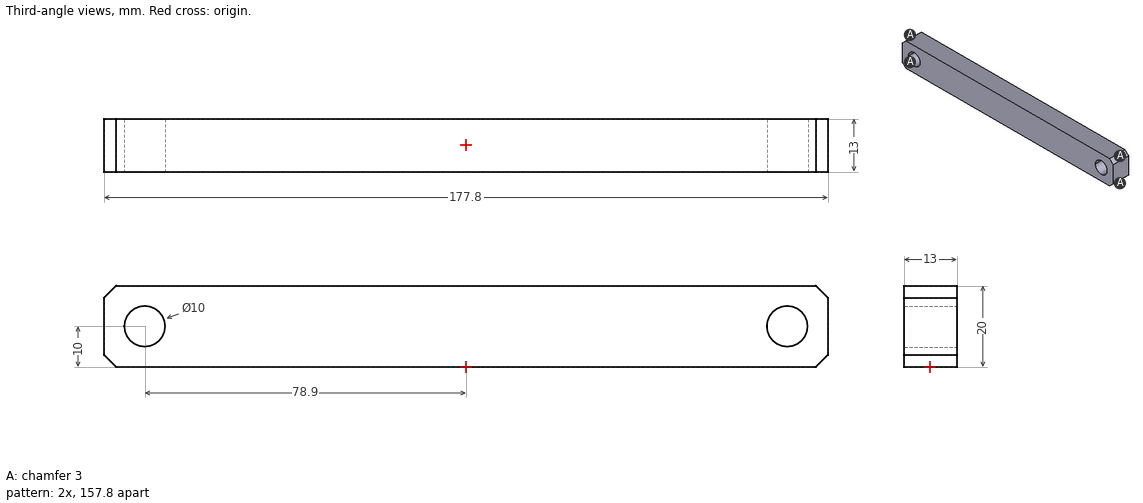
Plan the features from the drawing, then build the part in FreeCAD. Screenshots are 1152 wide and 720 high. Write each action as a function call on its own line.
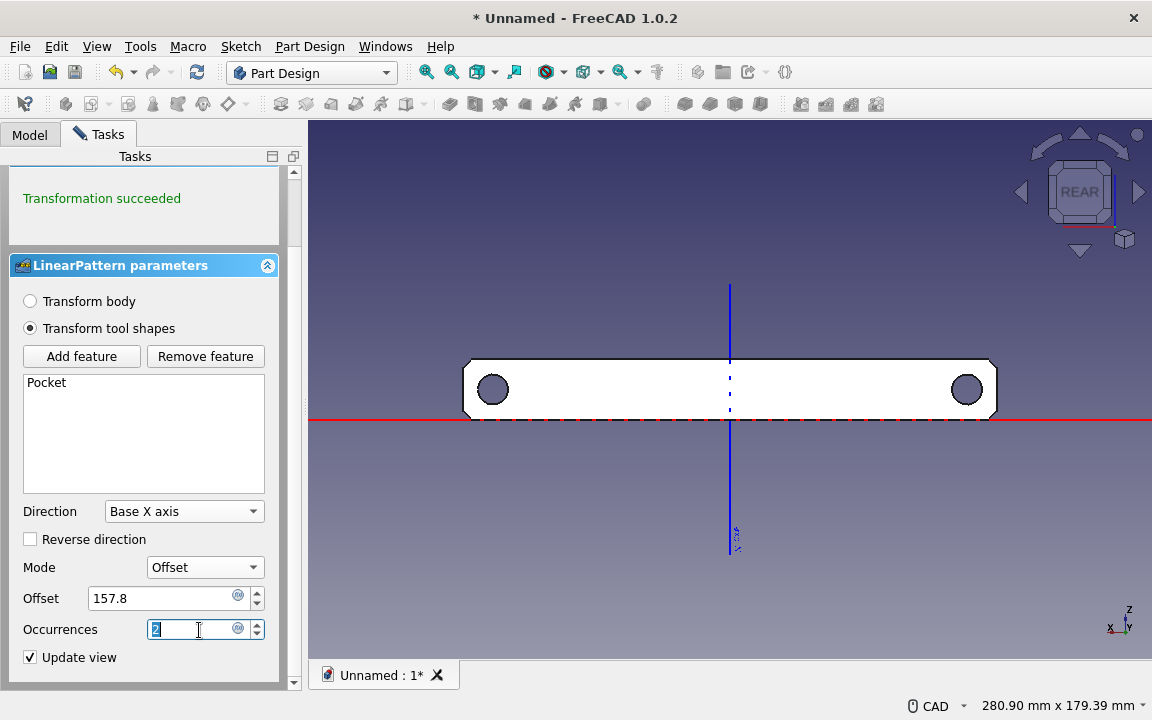
text(2)
key(Tab)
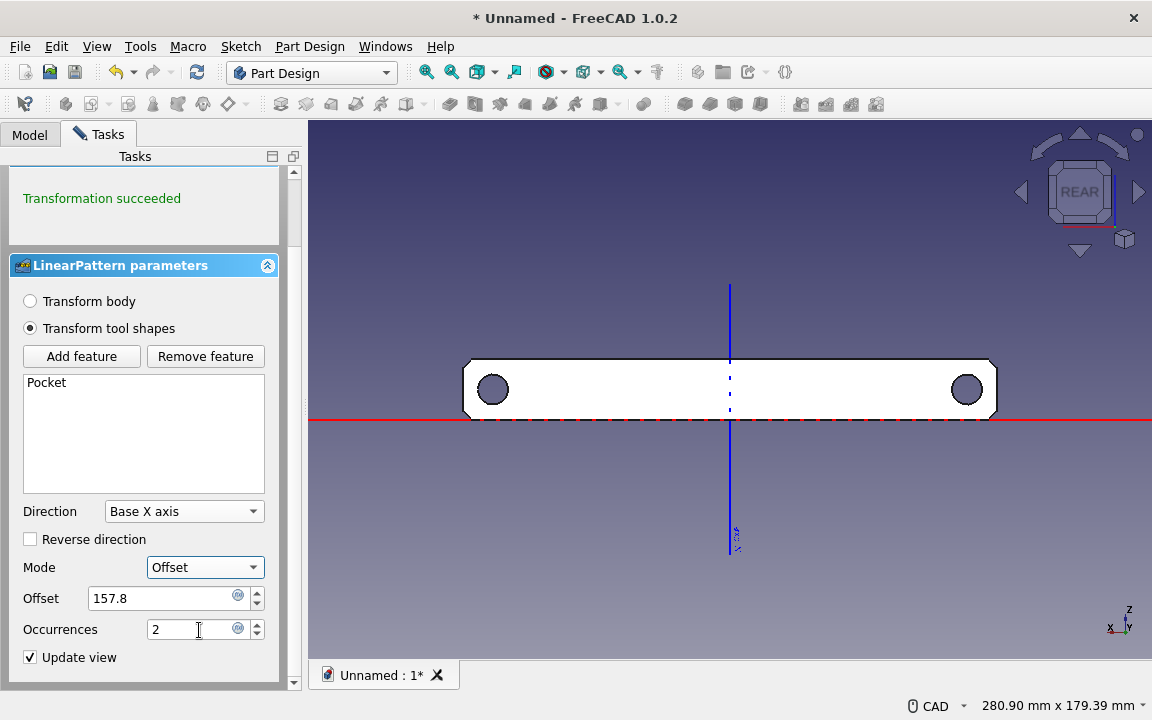
scroll(294, 428, up, 3)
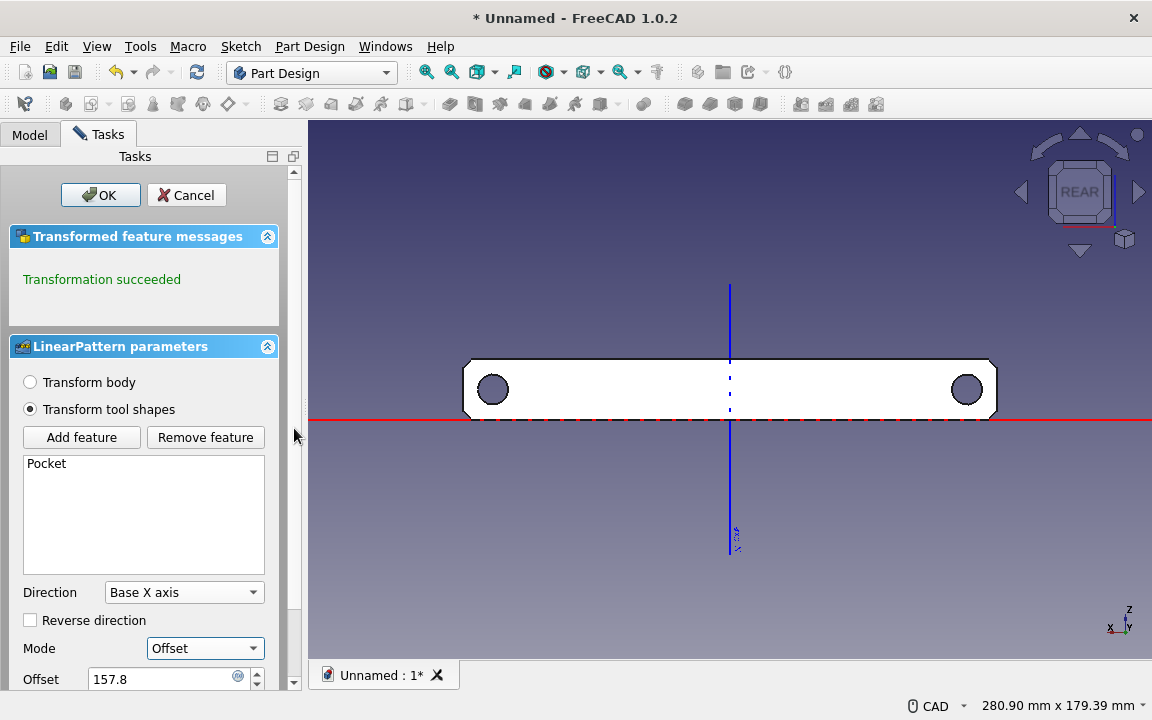
click(101, 195)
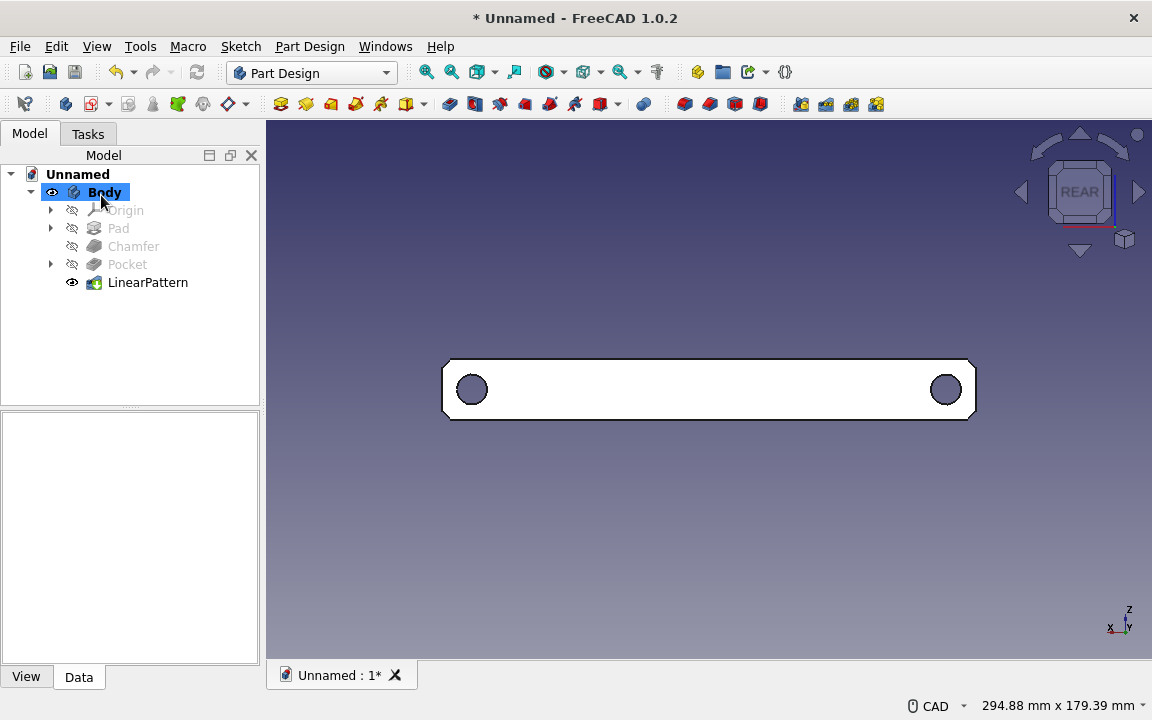
key(0)